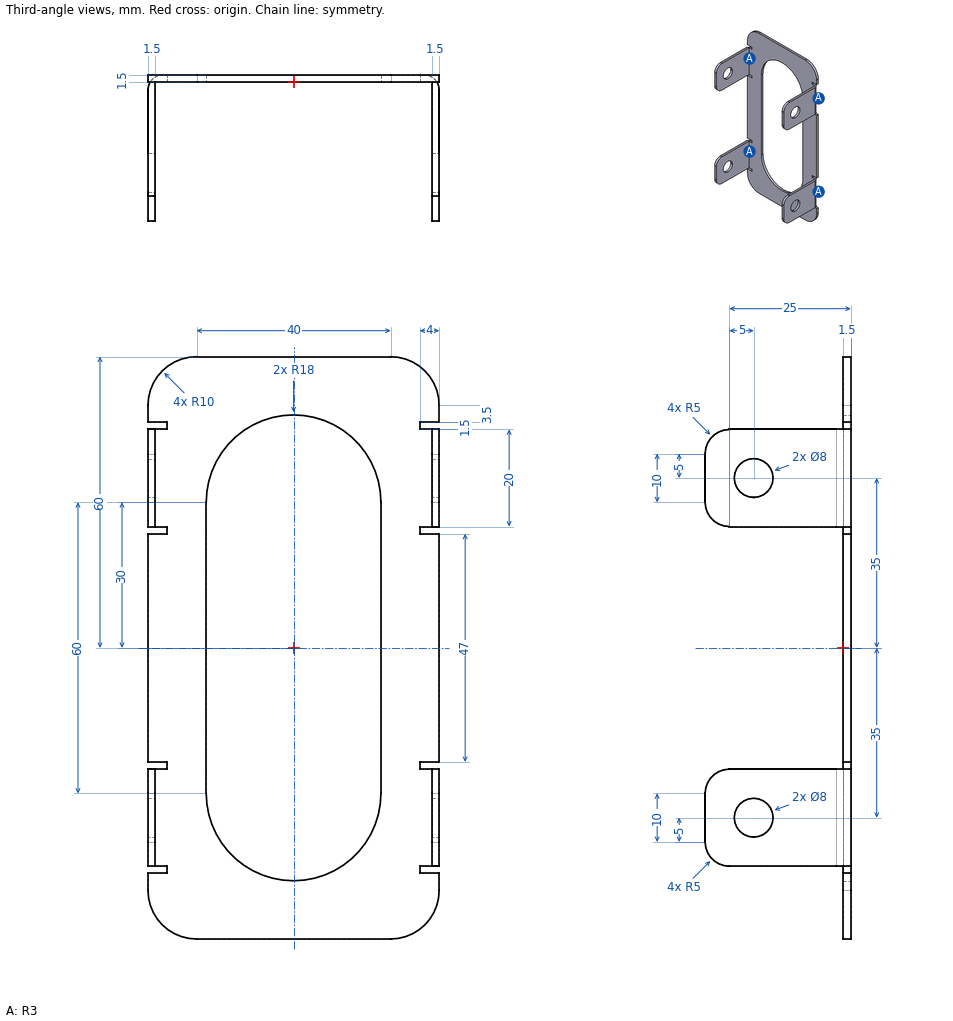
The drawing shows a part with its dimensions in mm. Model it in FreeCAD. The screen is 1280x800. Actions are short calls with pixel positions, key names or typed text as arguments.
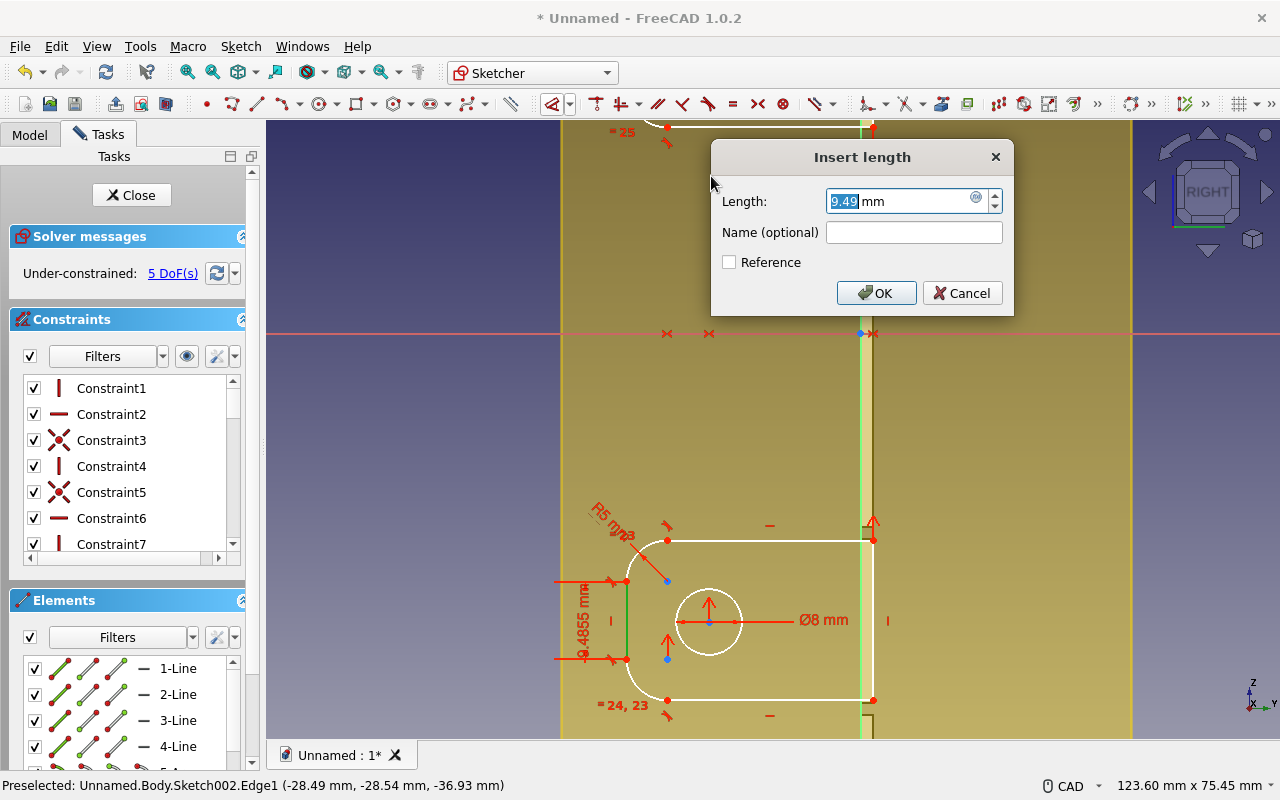
text(10)
key(Return)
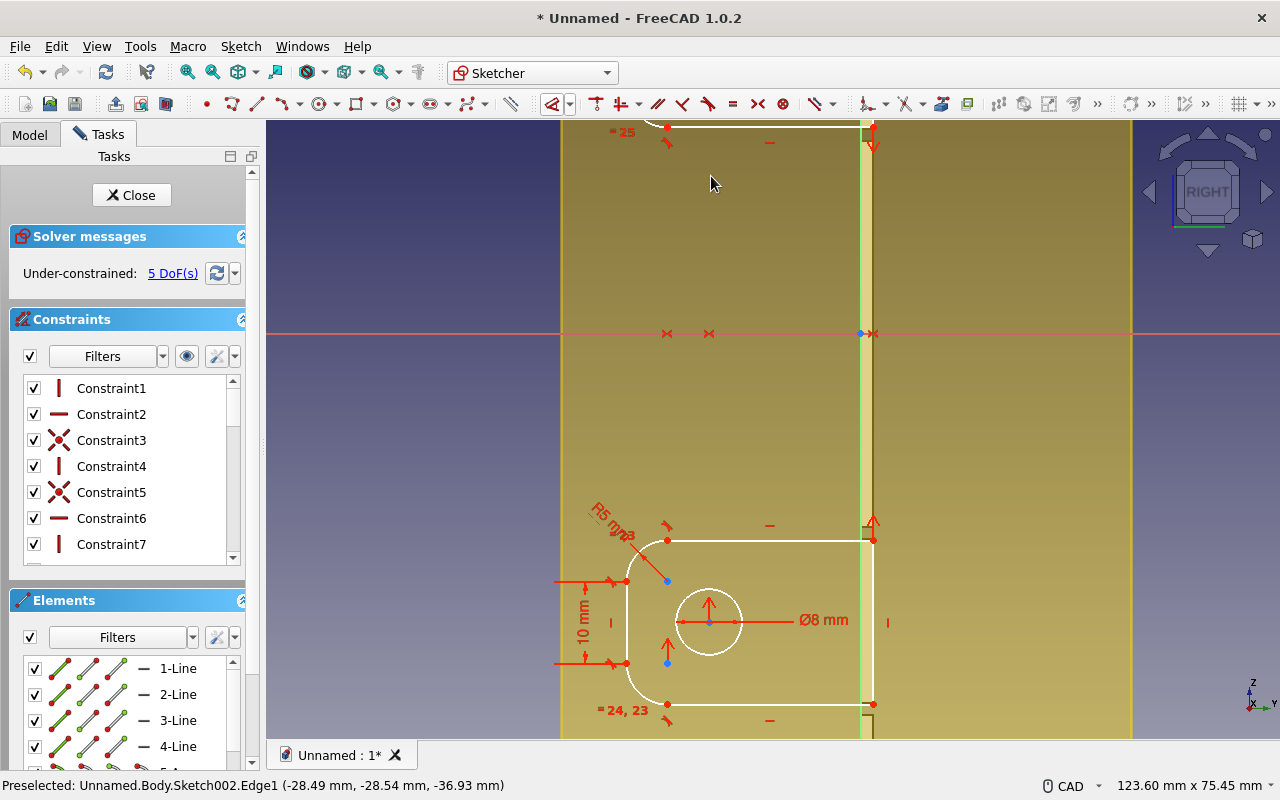
click(729, 540)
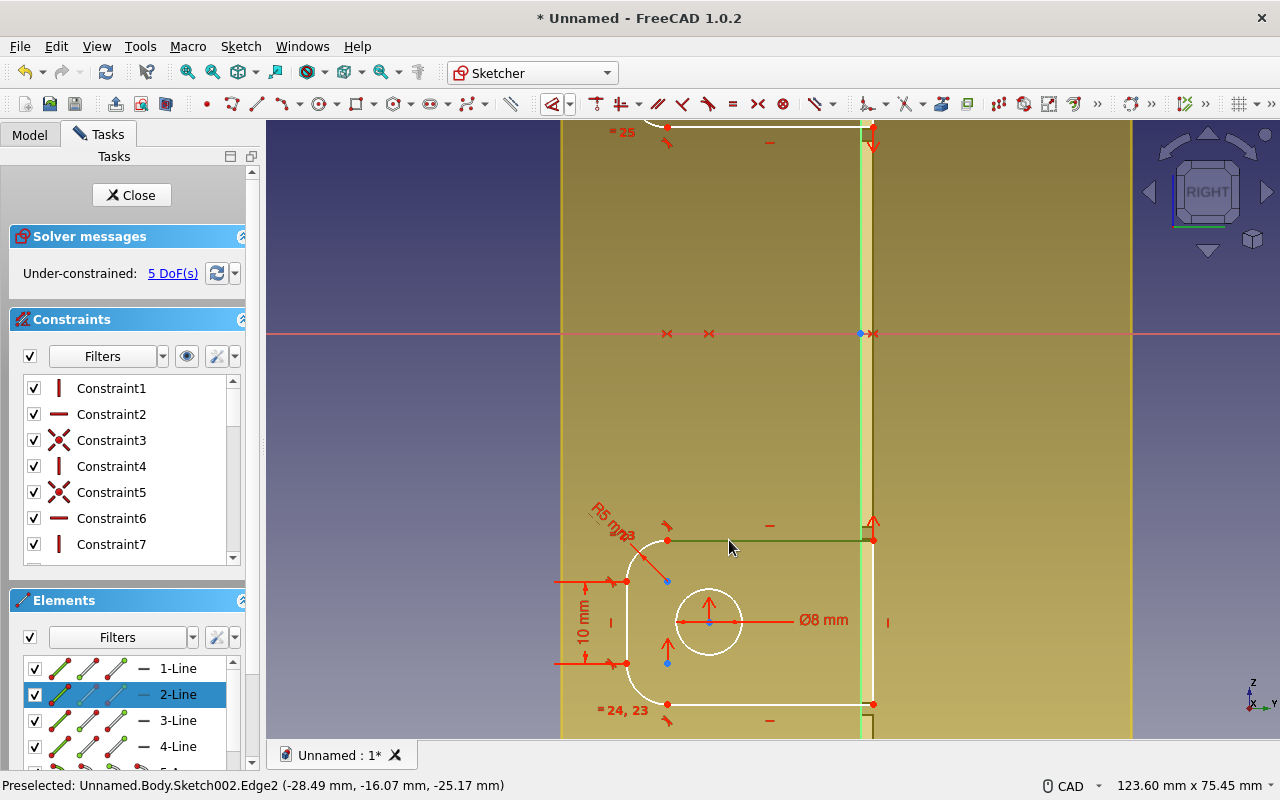
key(l)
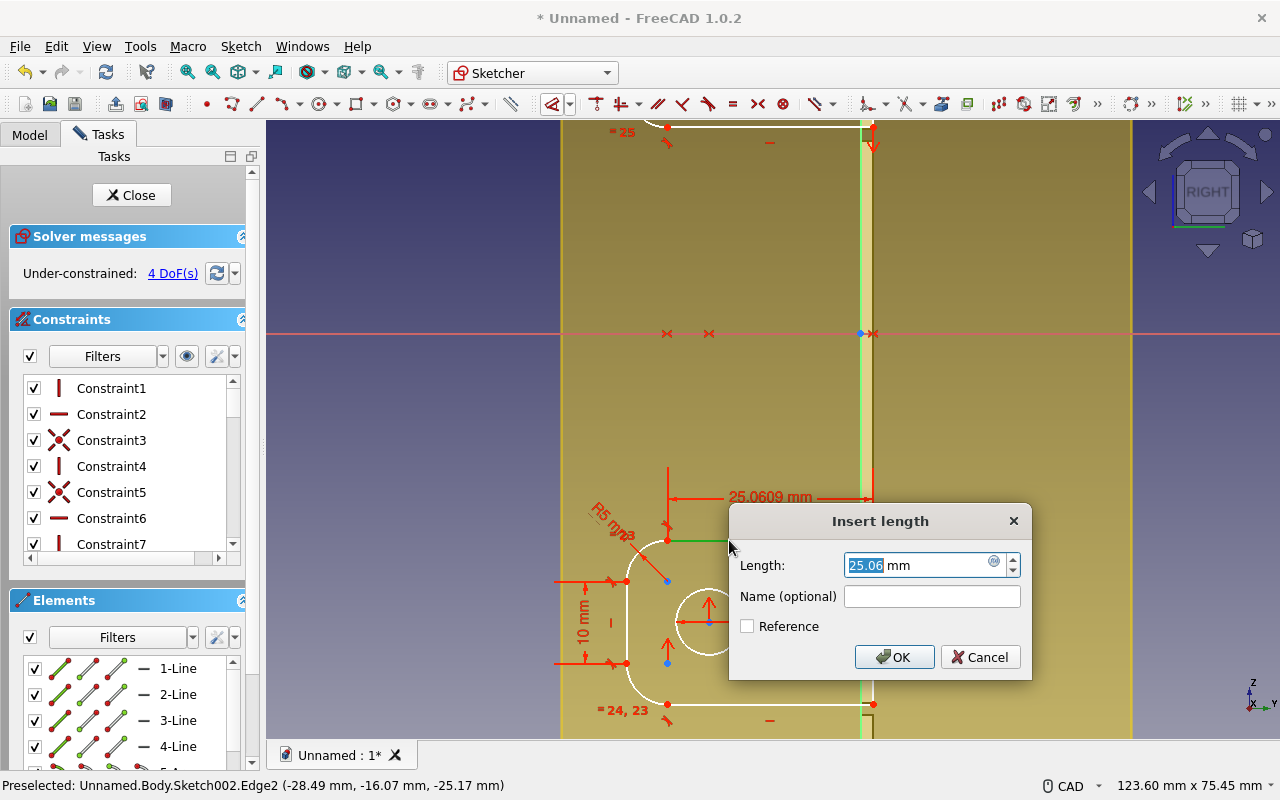
text(25)
key(Return)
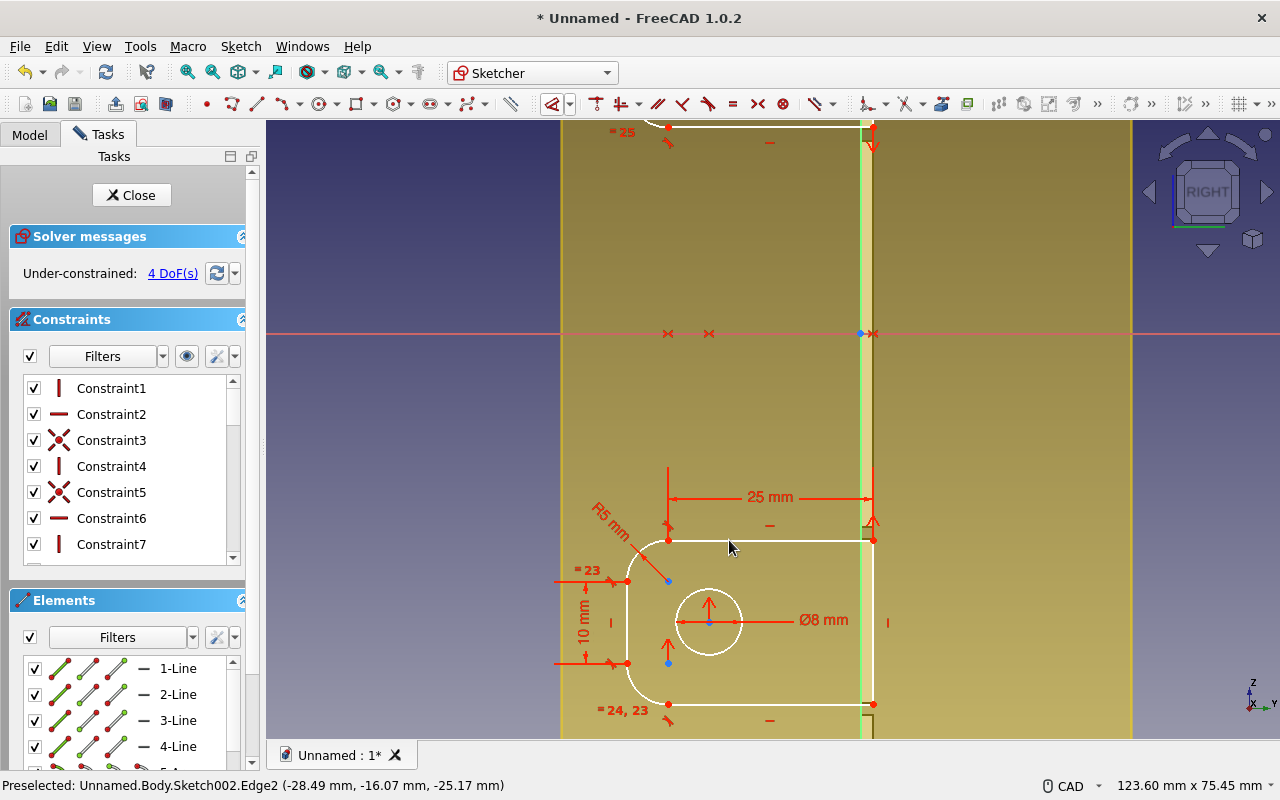
click(709, 622)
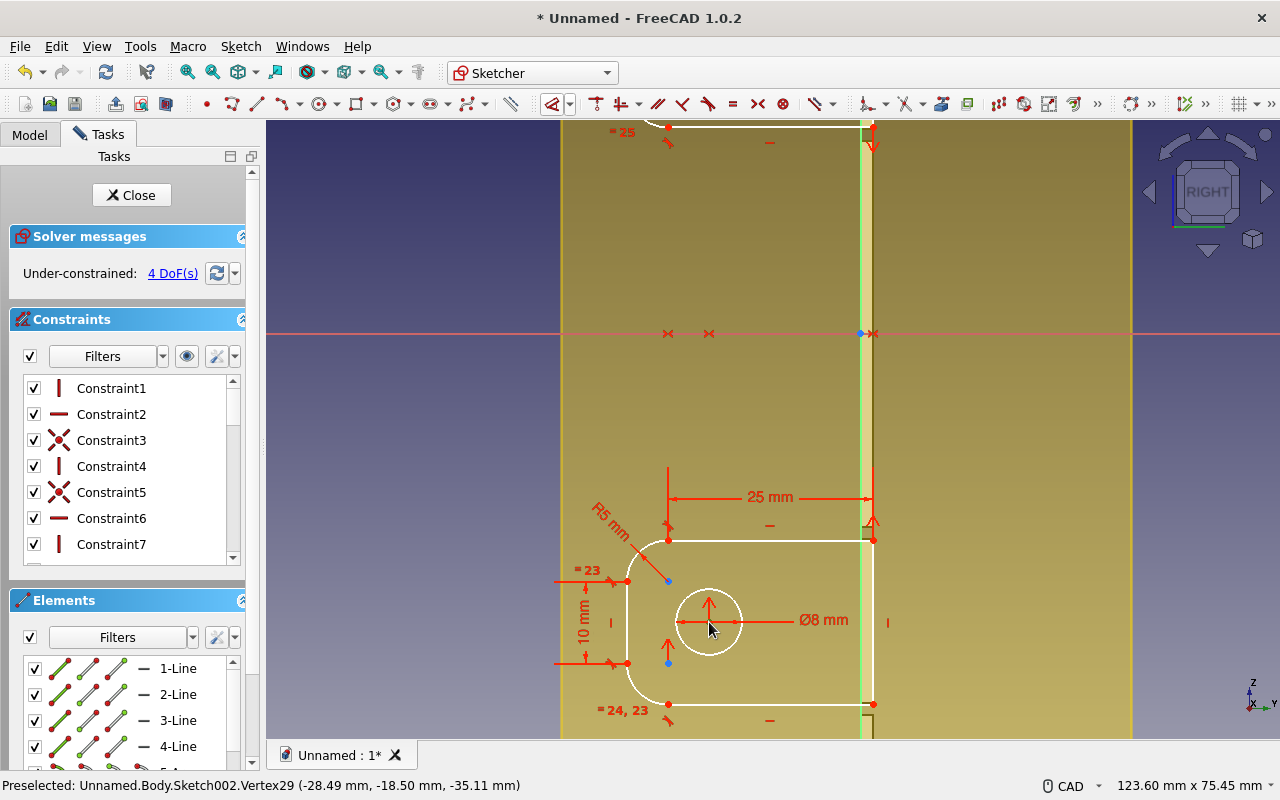
click(570, 104)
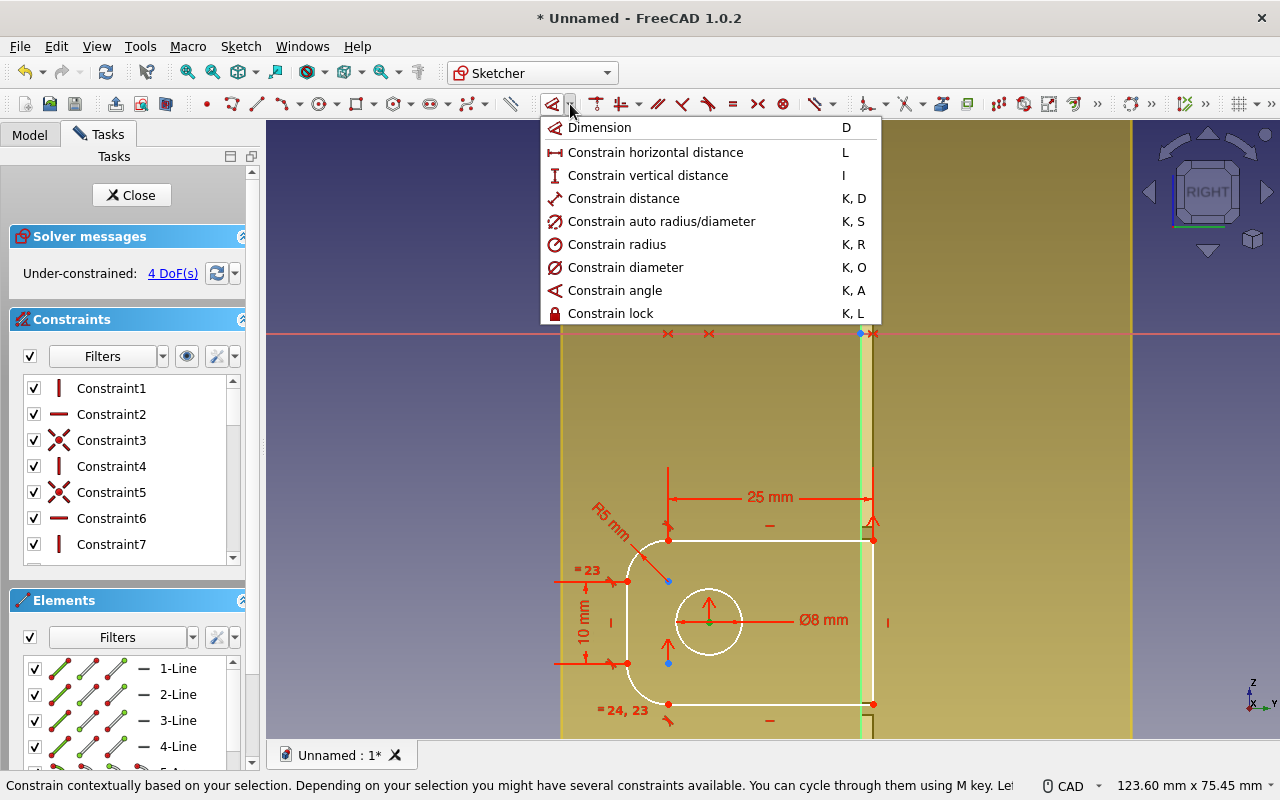
click(711, 176)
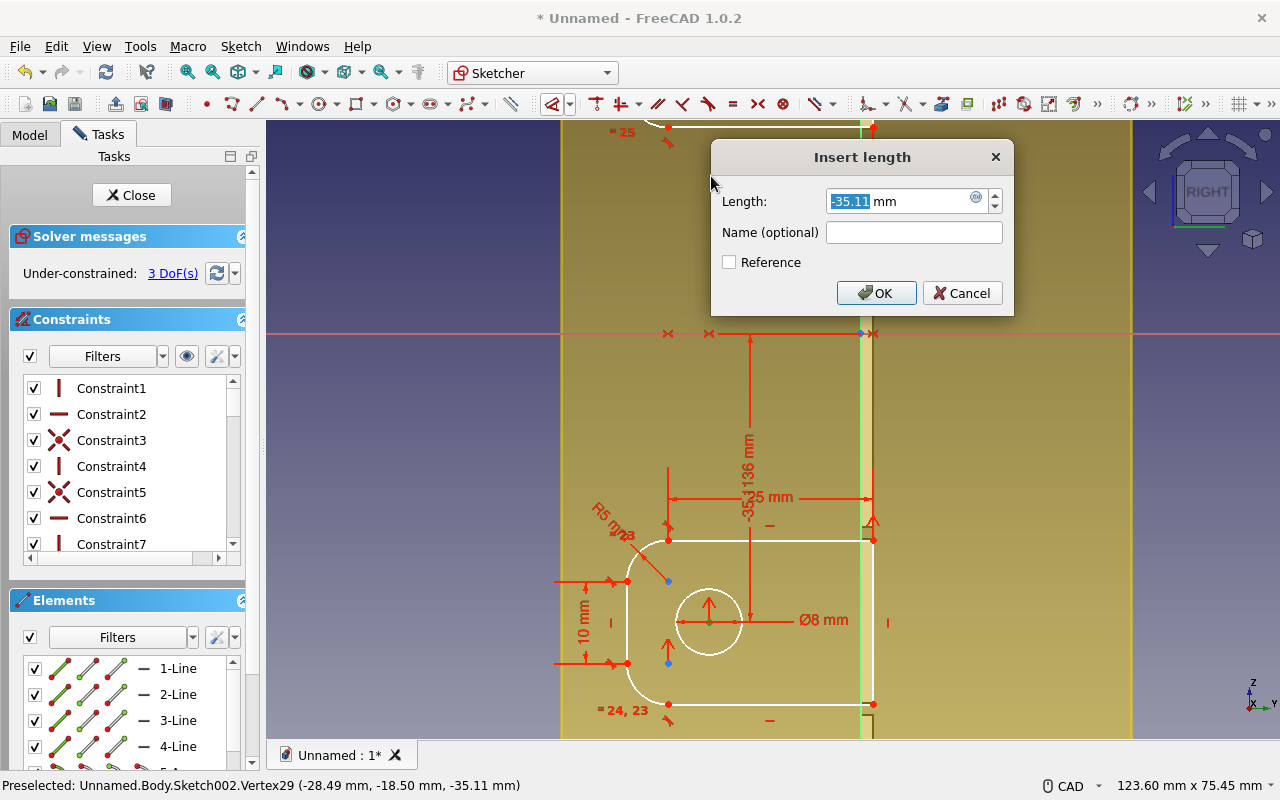
text(-35)
key(Return)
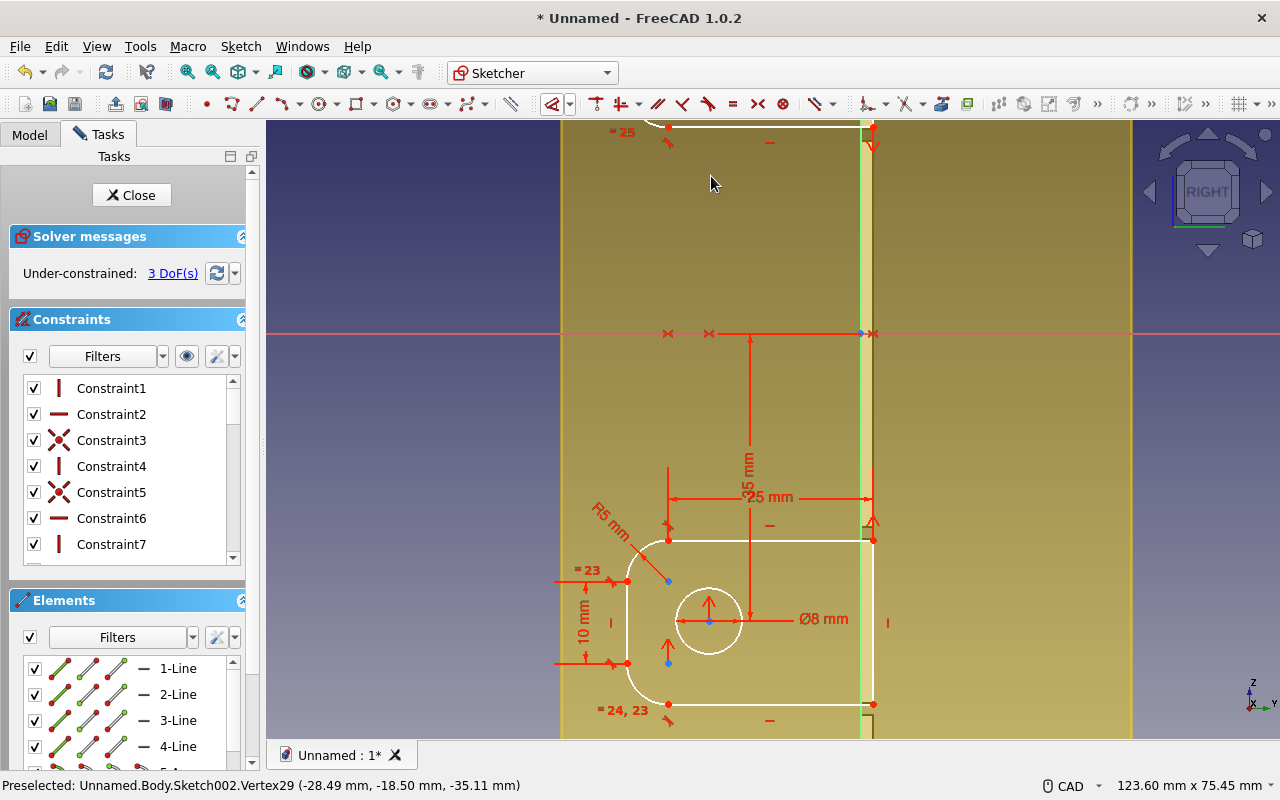
click(668, 540)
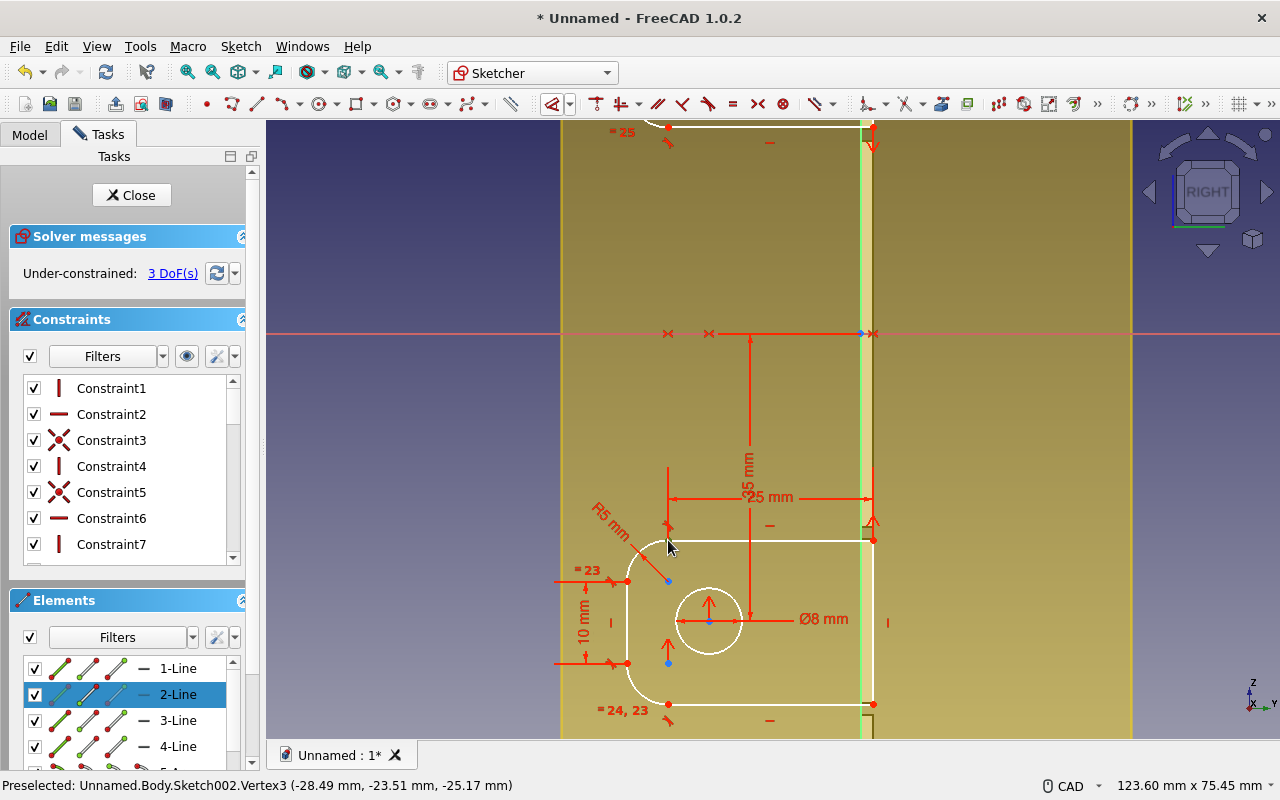
click(709, 621)